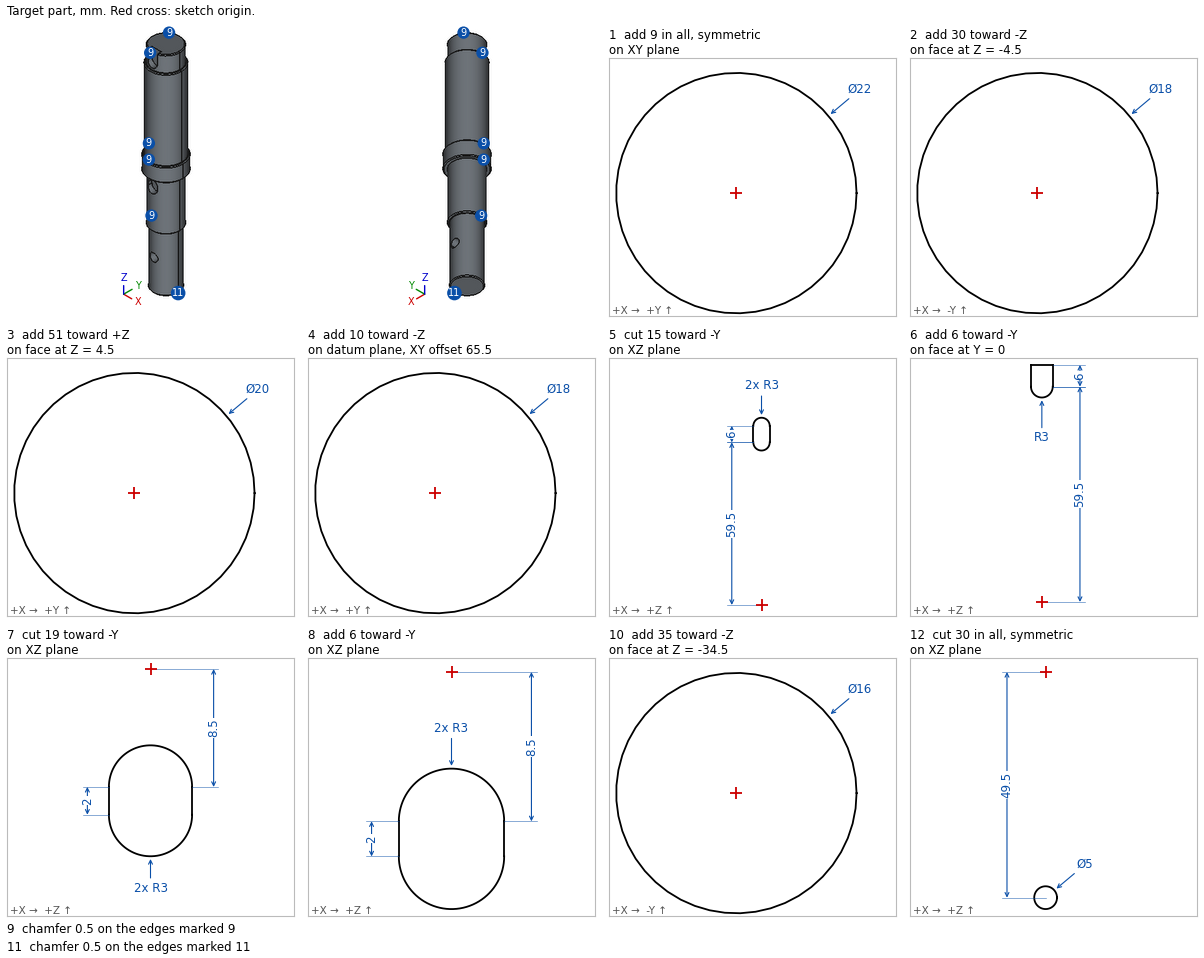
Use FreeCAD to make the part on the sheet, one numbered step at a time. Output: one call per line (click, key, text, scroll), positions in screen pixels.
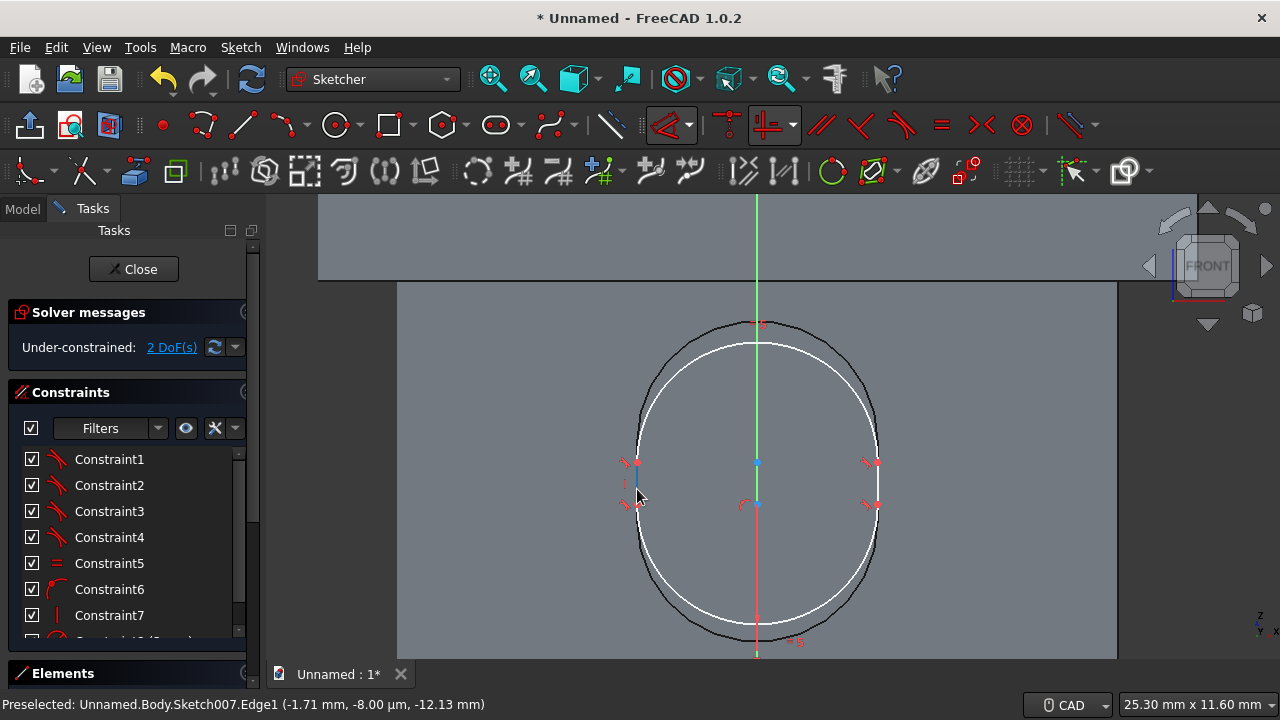
click(637, 488)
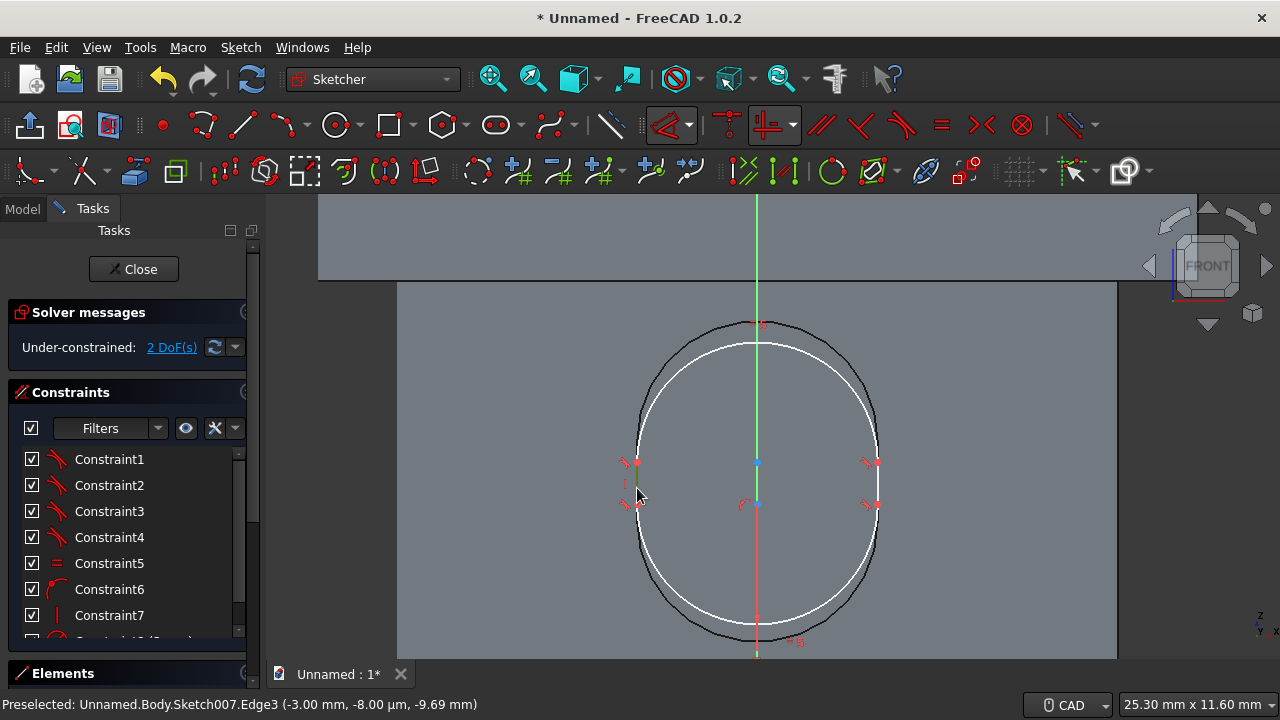
click(692, 126)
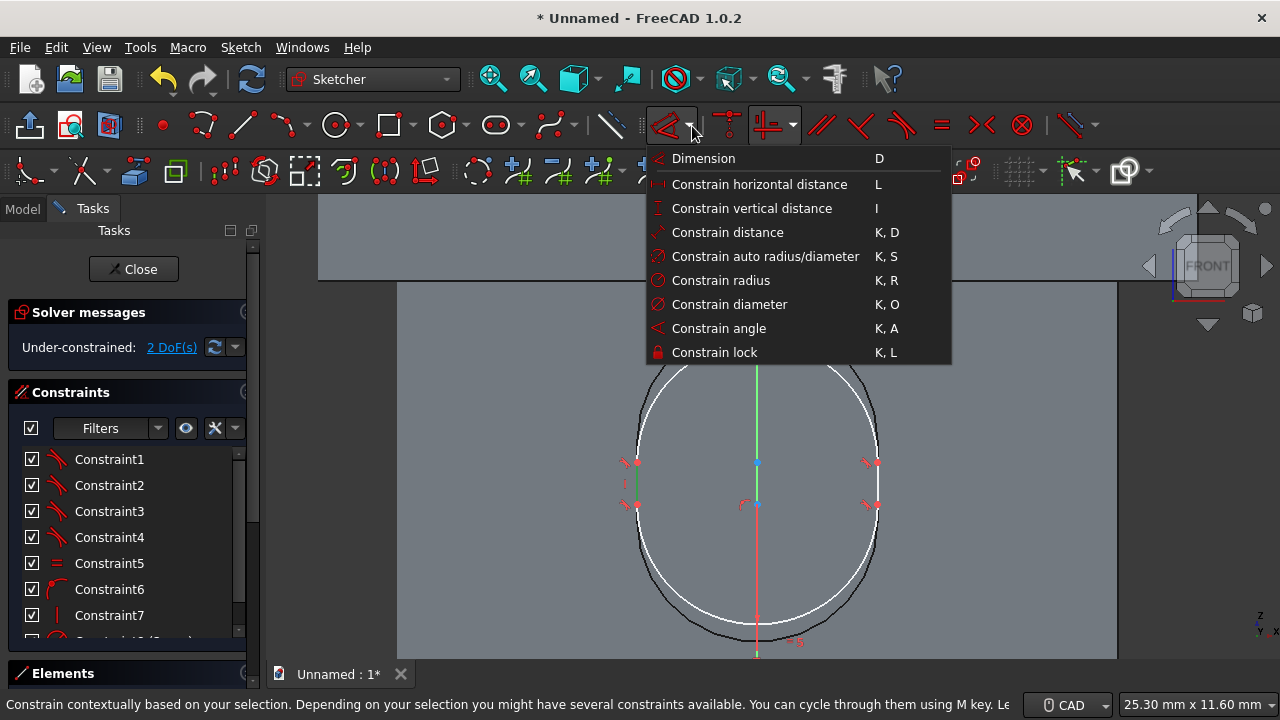
click(799, 208)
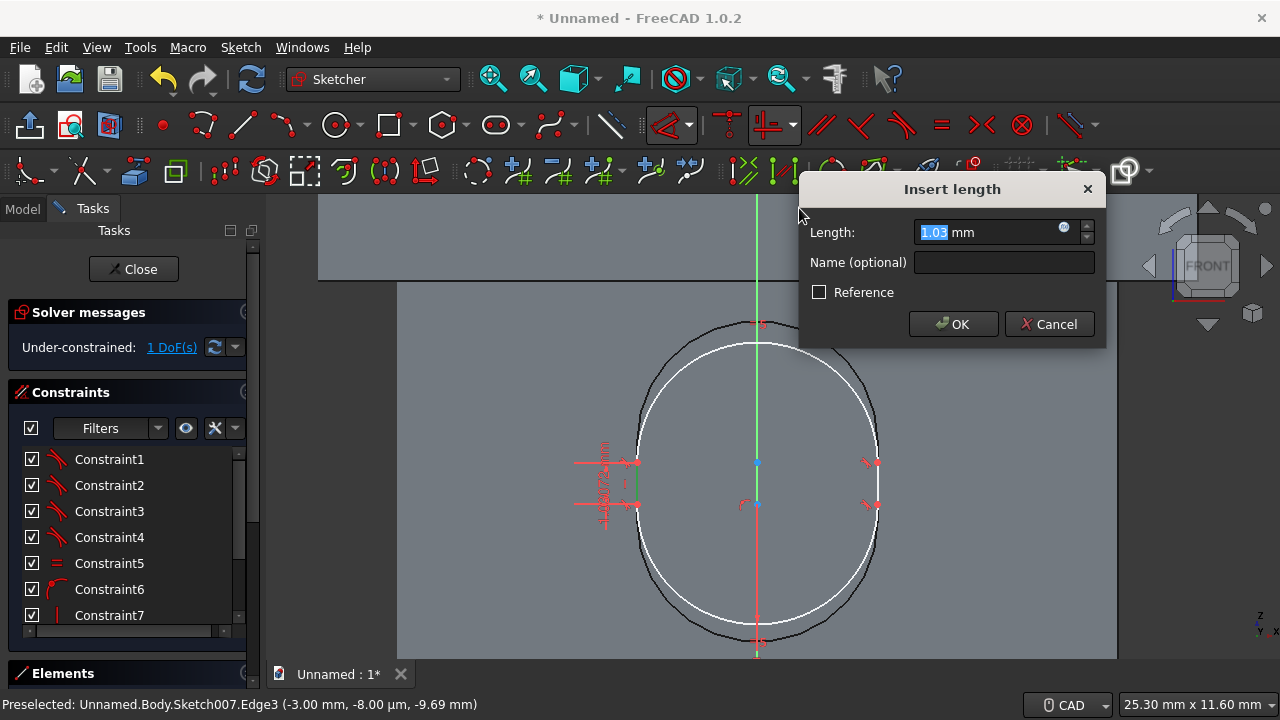
text(2)
key(Return)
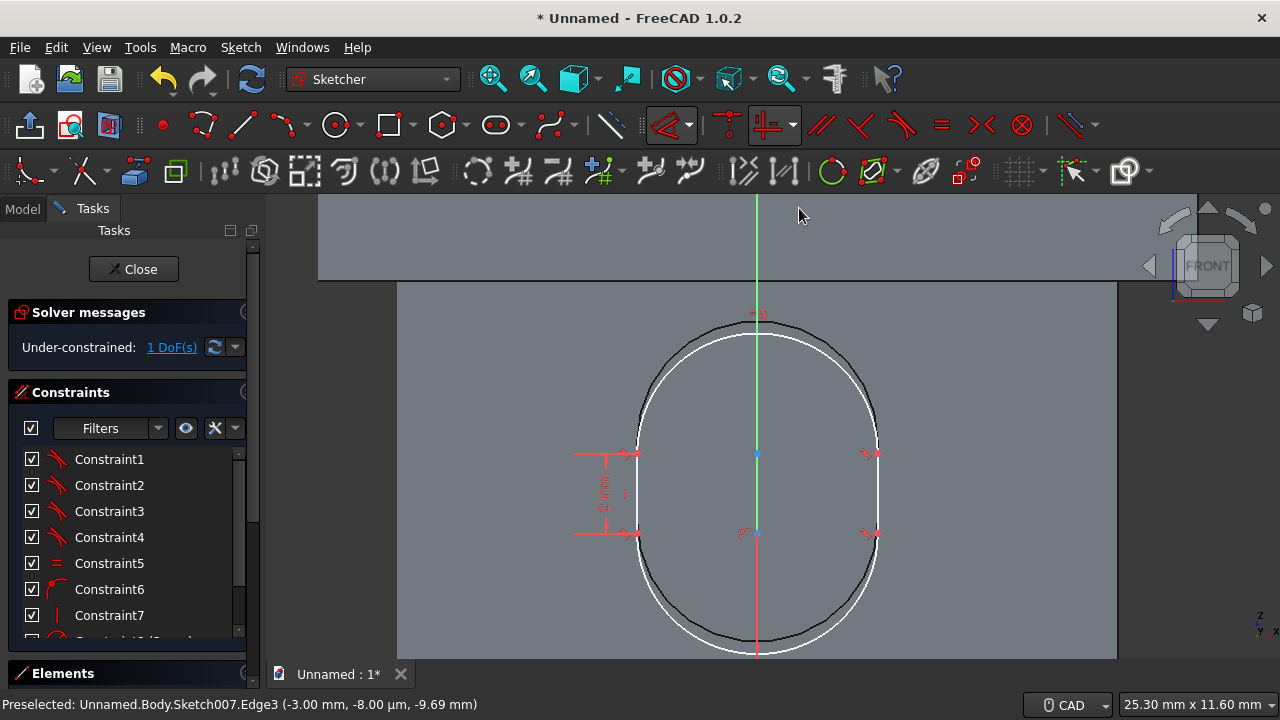
click(878, 454)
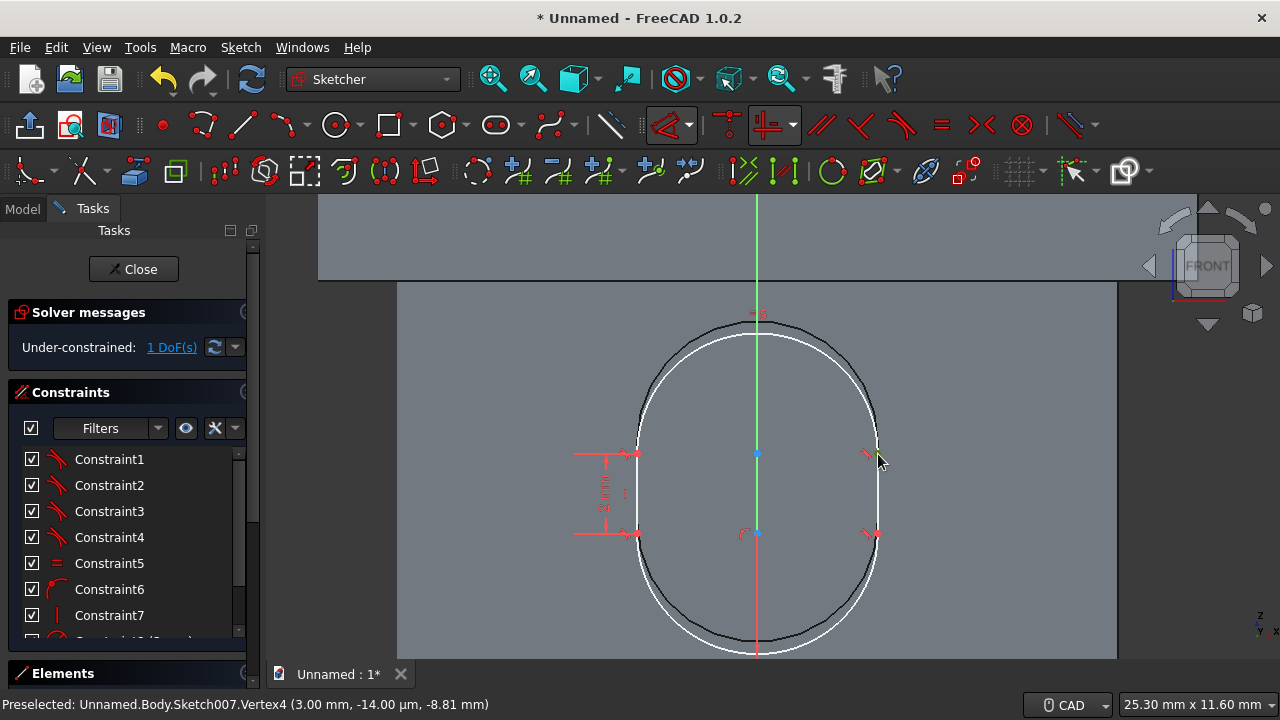
key(i)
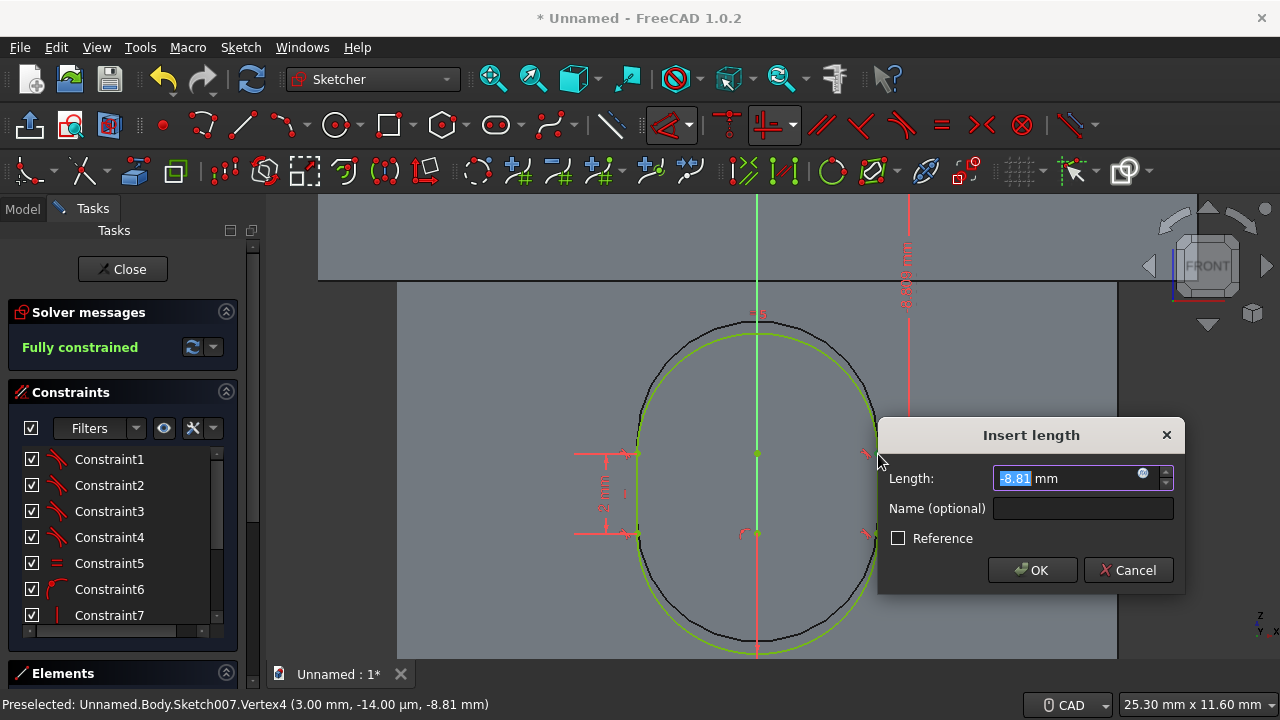
text(-8.5)
key(Return)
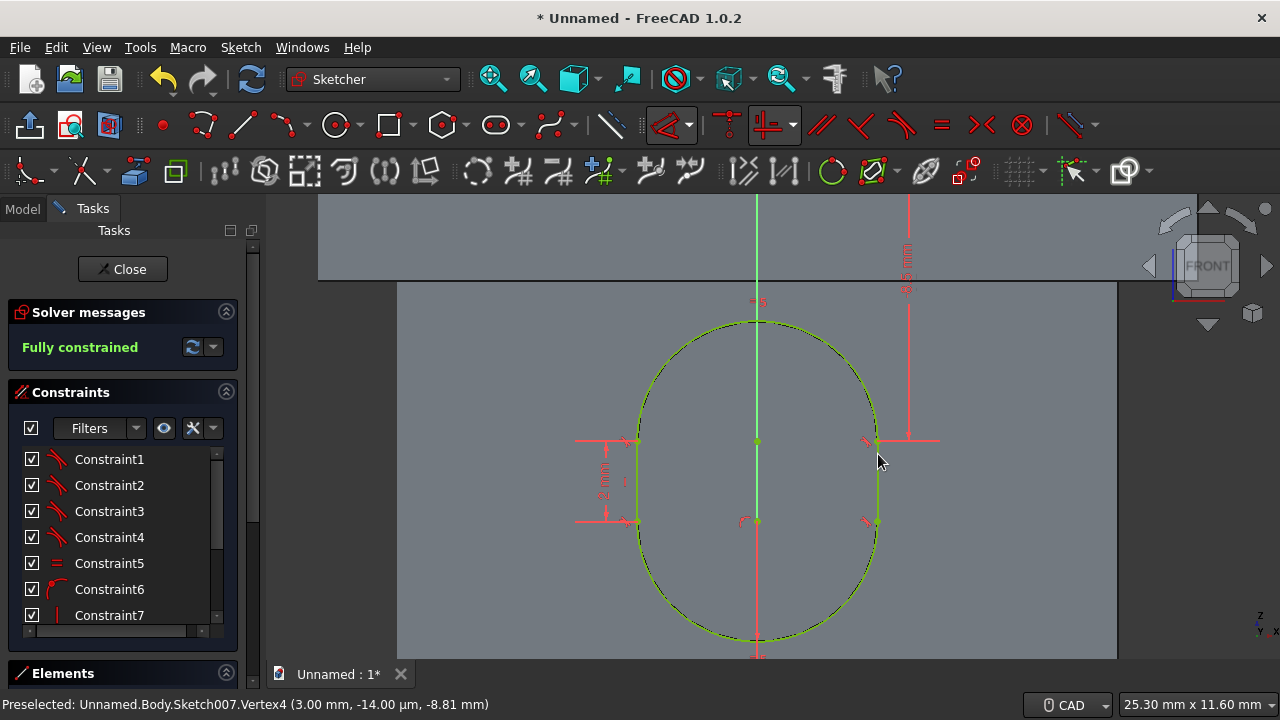
click(123, 269)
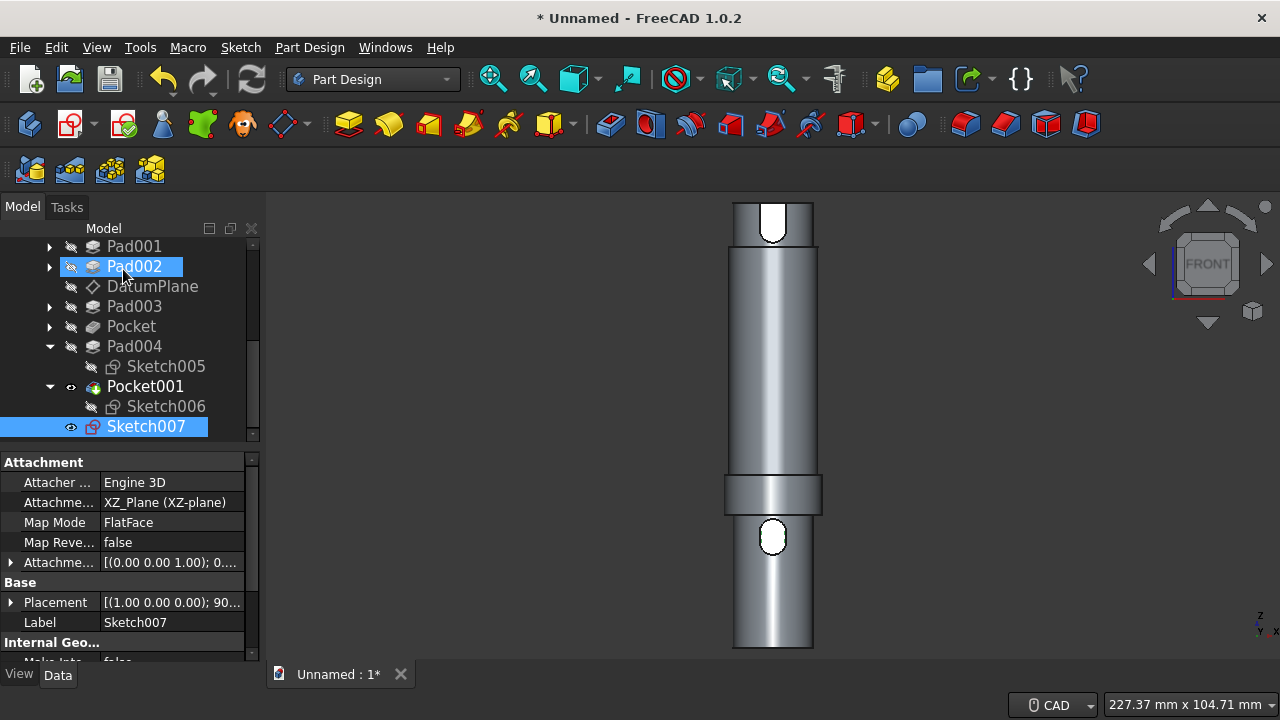
click(350, 124)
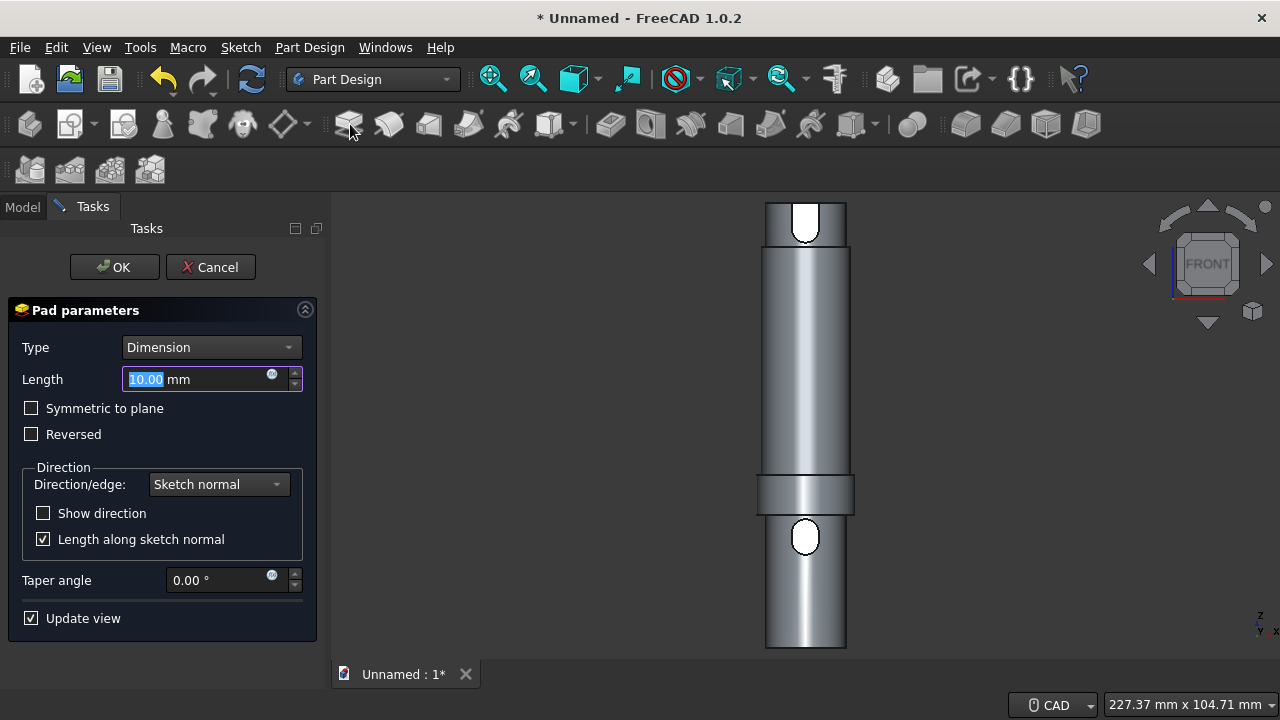
text(6)
key(Tab)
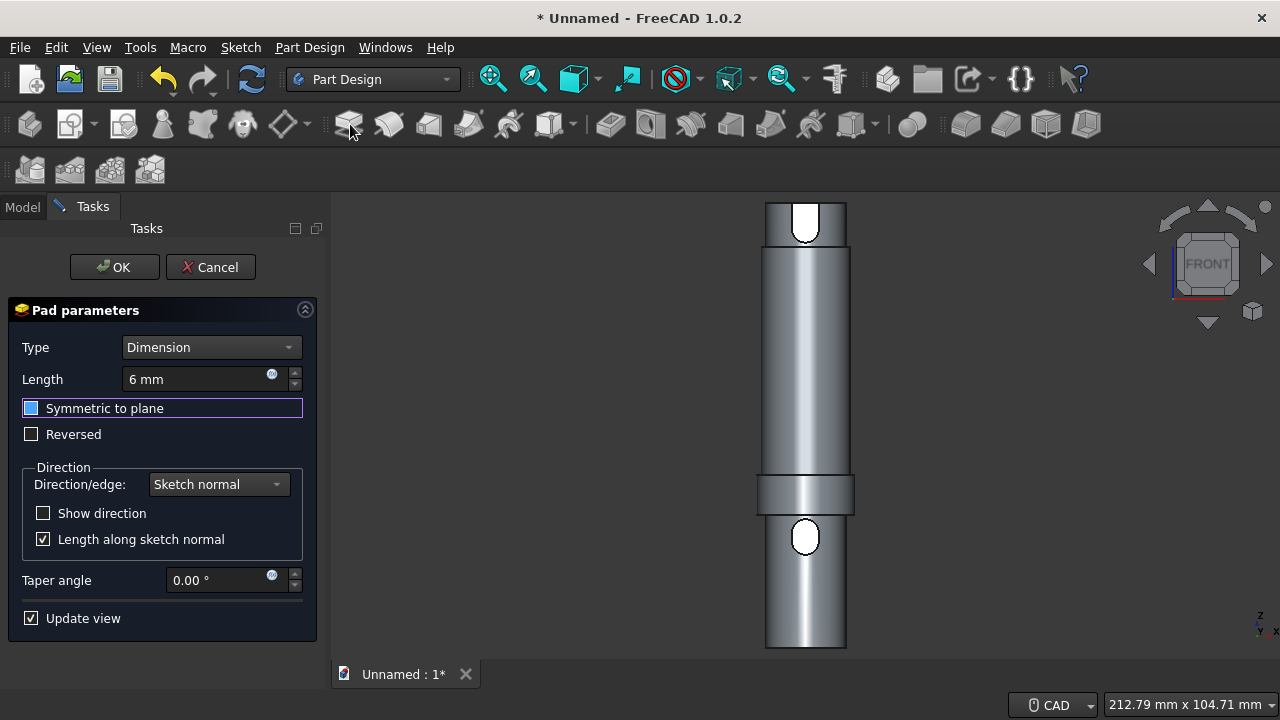
click(115, 267)